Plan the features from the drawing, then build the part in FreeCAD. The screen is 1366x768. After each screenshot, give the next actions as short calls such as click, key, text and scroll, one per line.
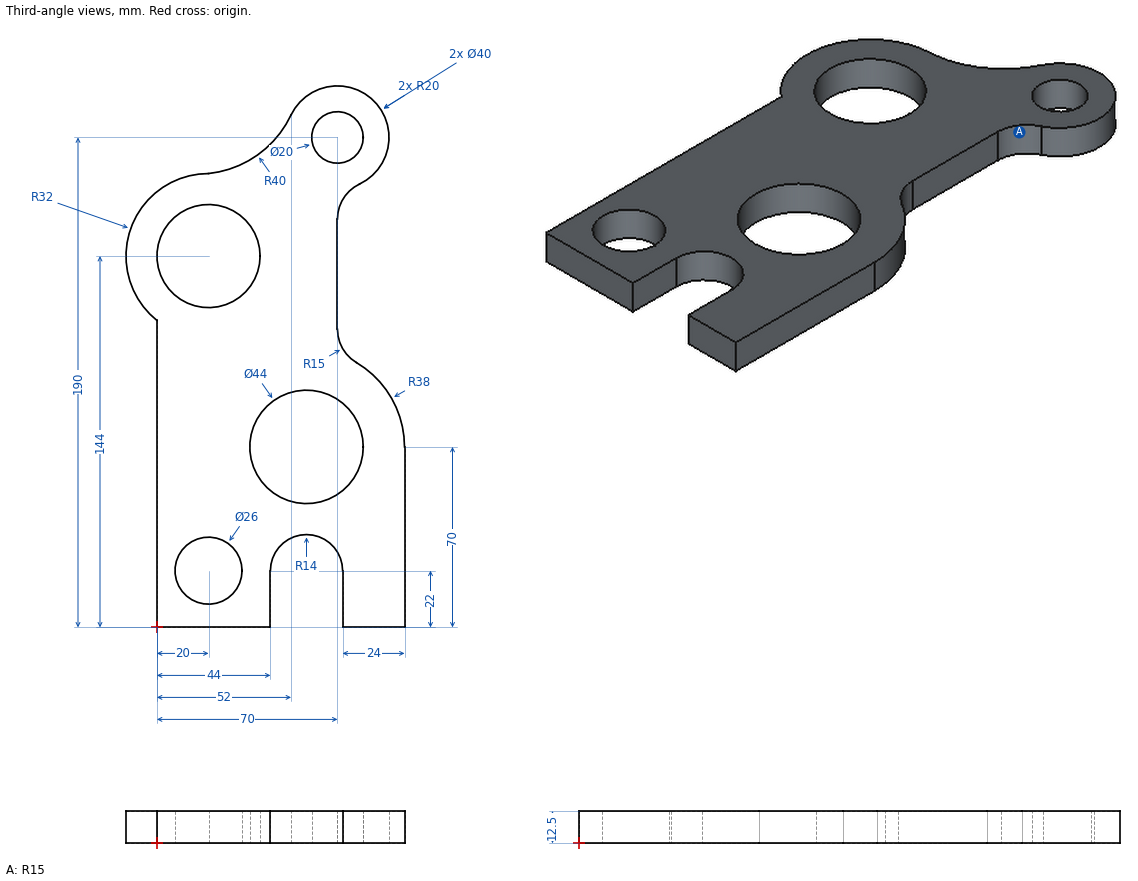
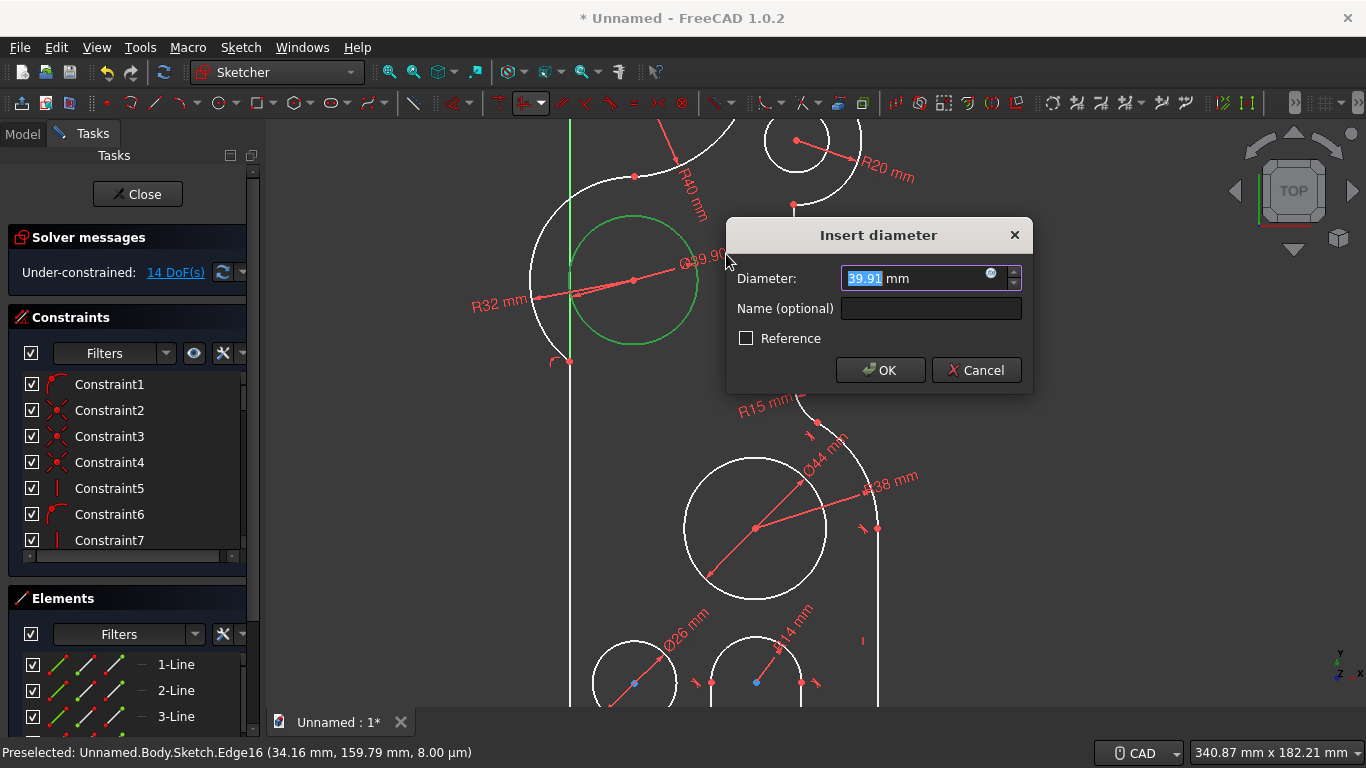
text(40)
key(Return)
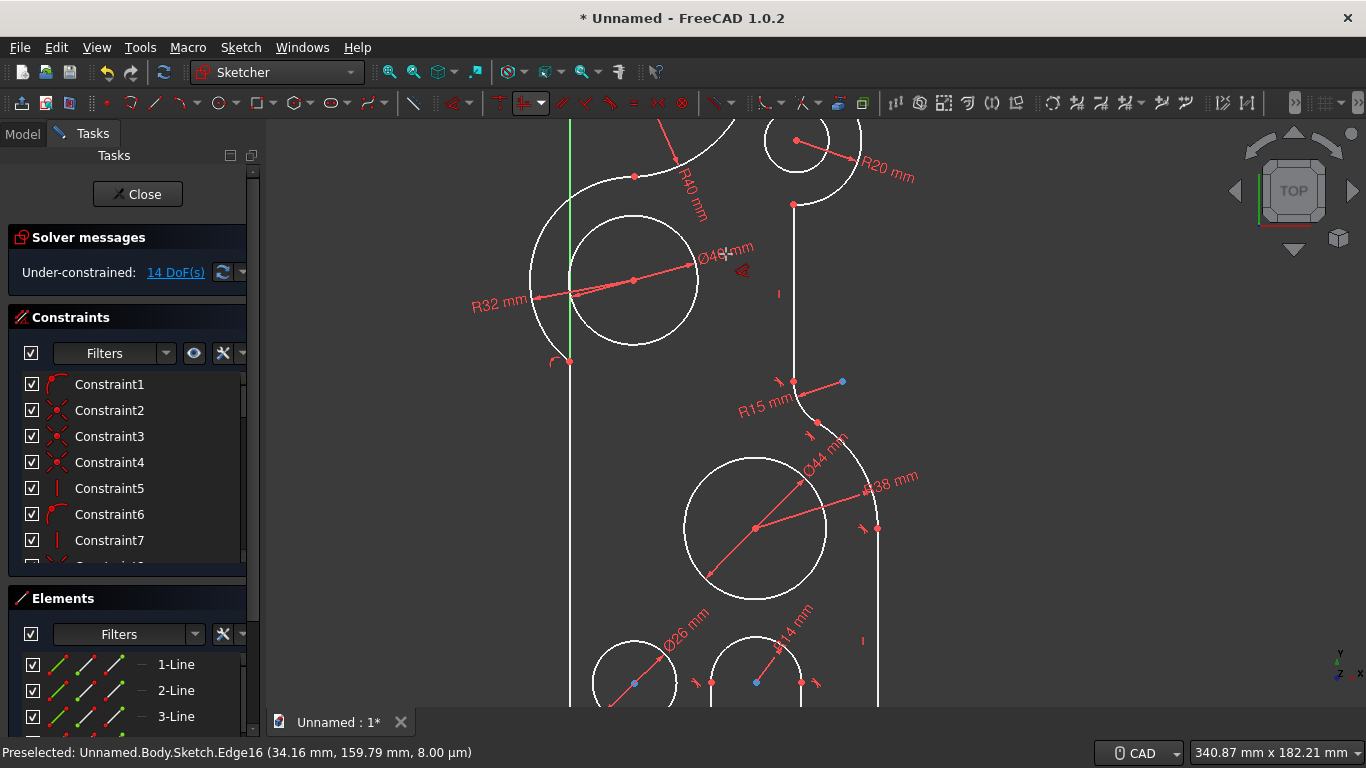
click(774, 163)
click(735, 158)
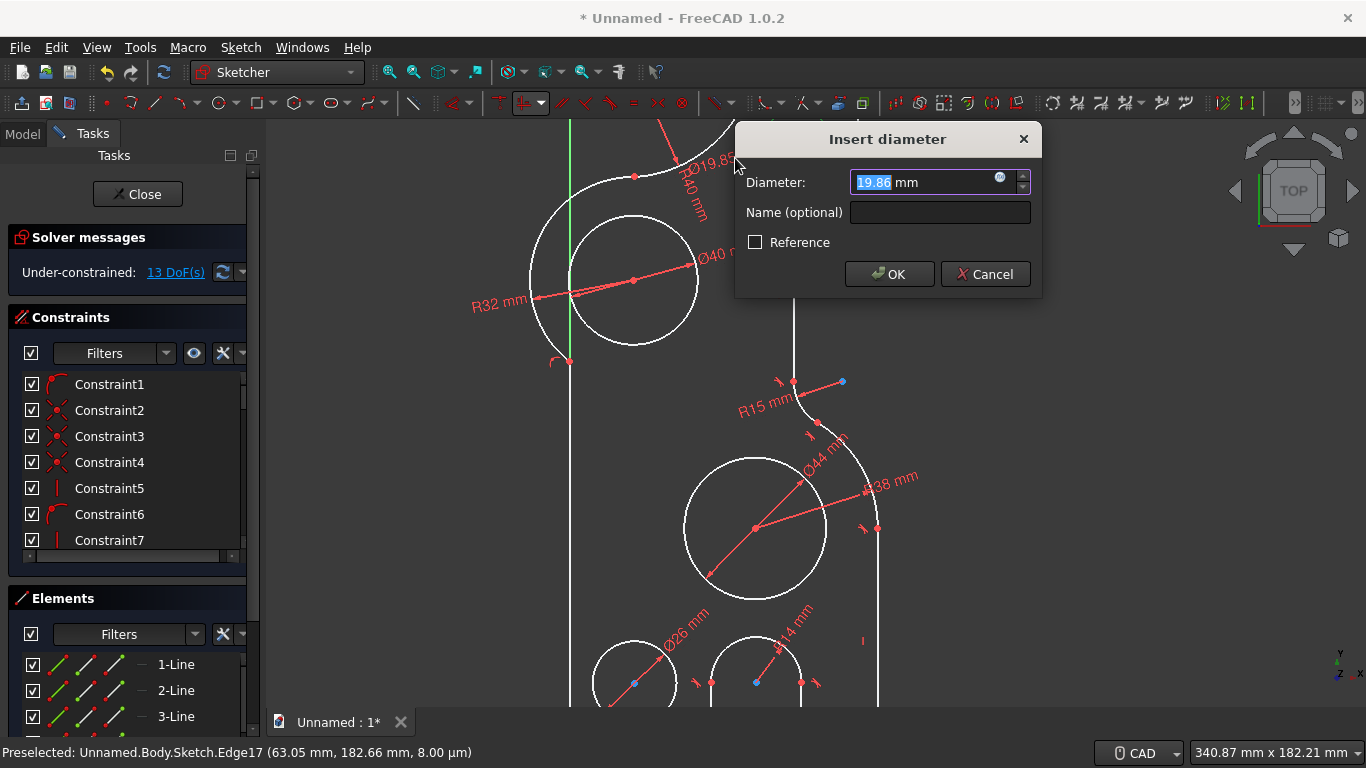
text(20)
key(Return)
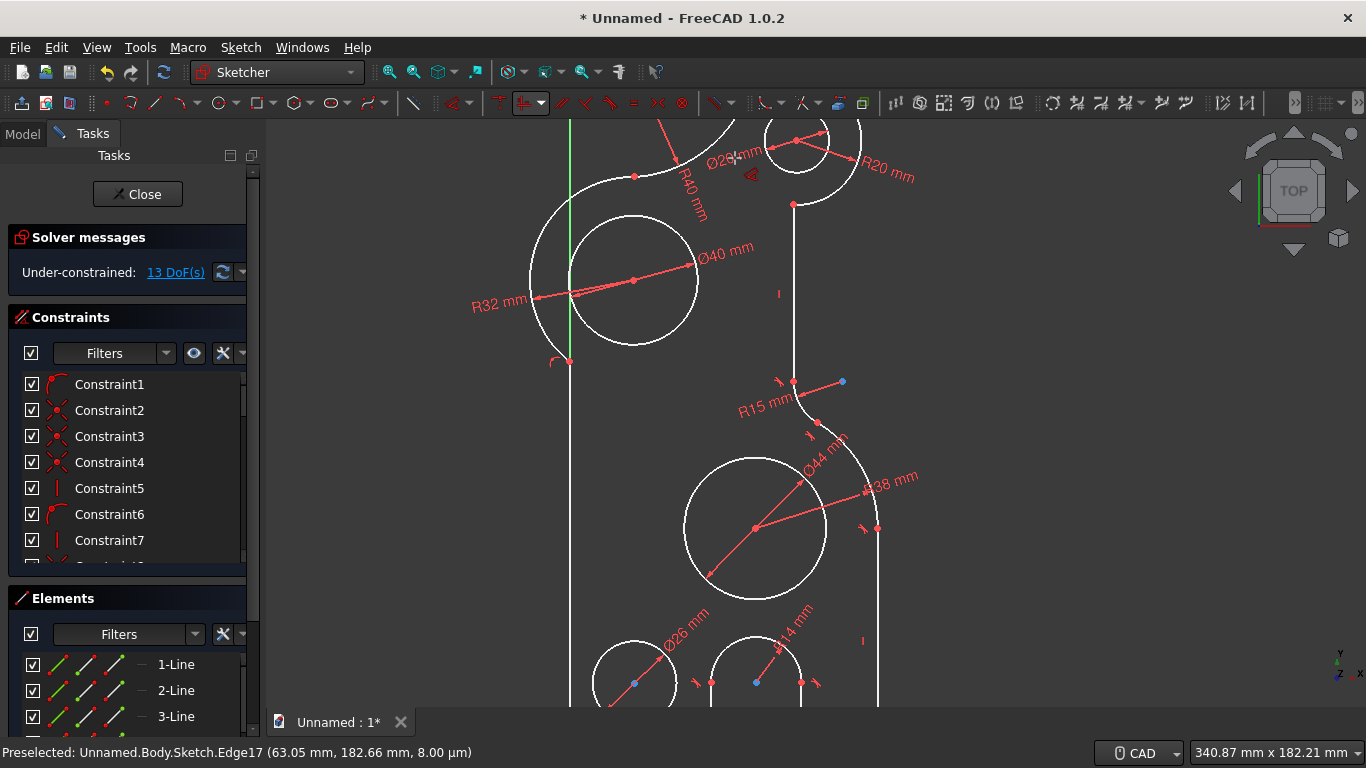
scroll(795, 395, down, 3)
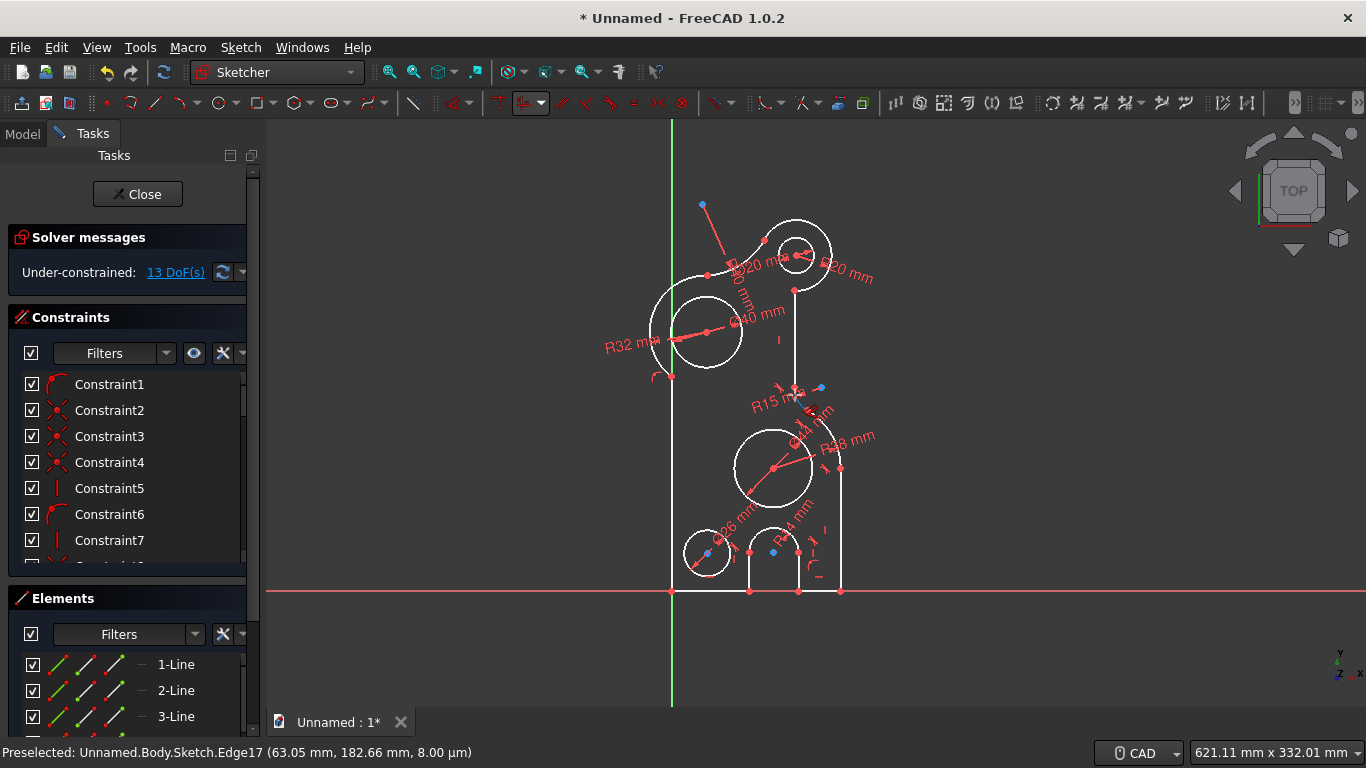
click(695, 591)
click(710, 625)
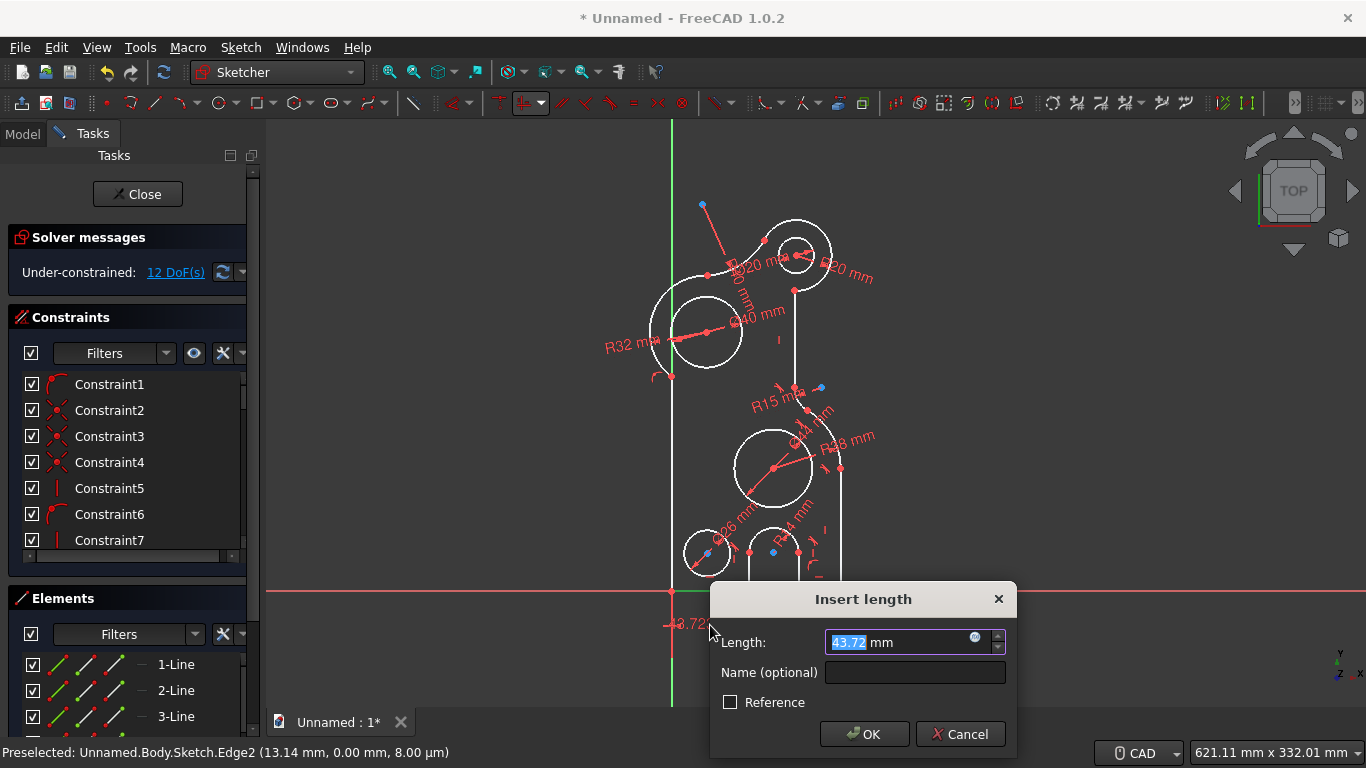
text(44)
key(Return)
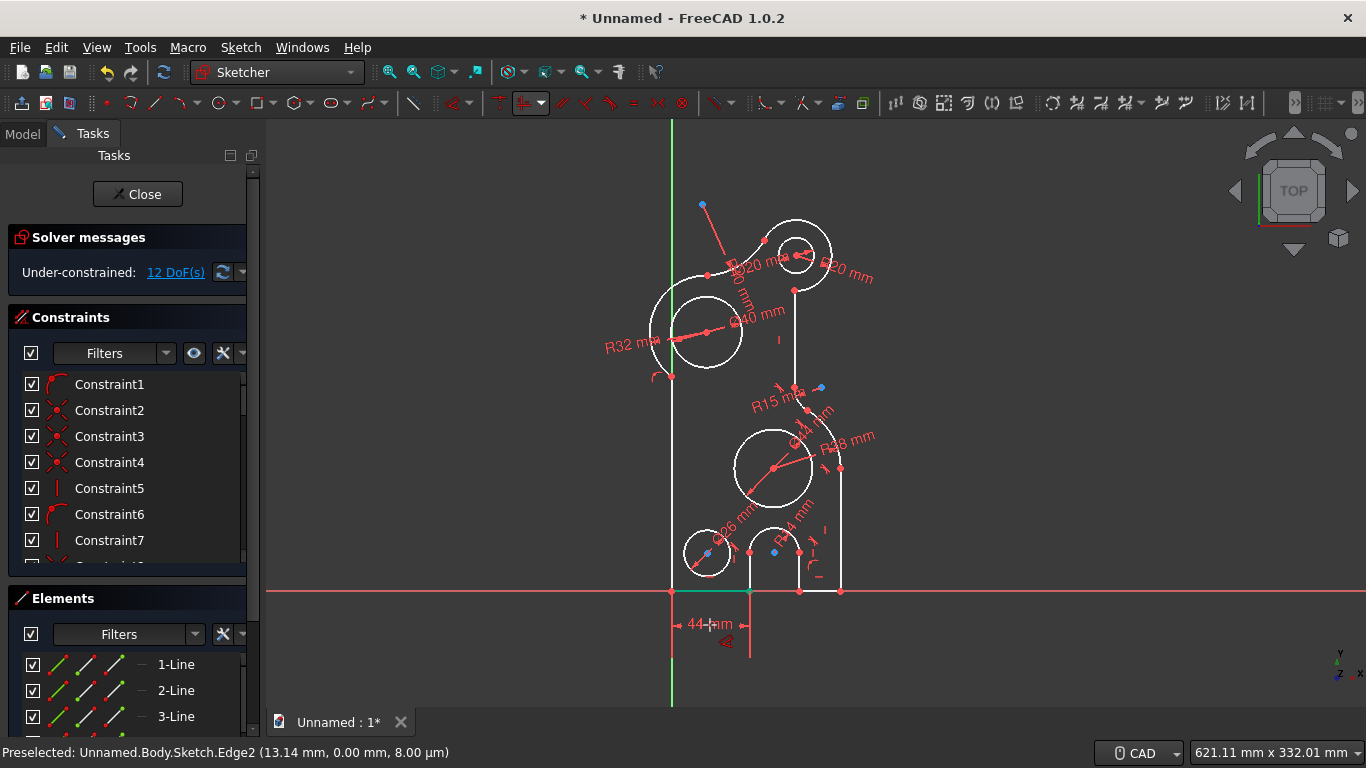
click(750, 580)
click(784, 572)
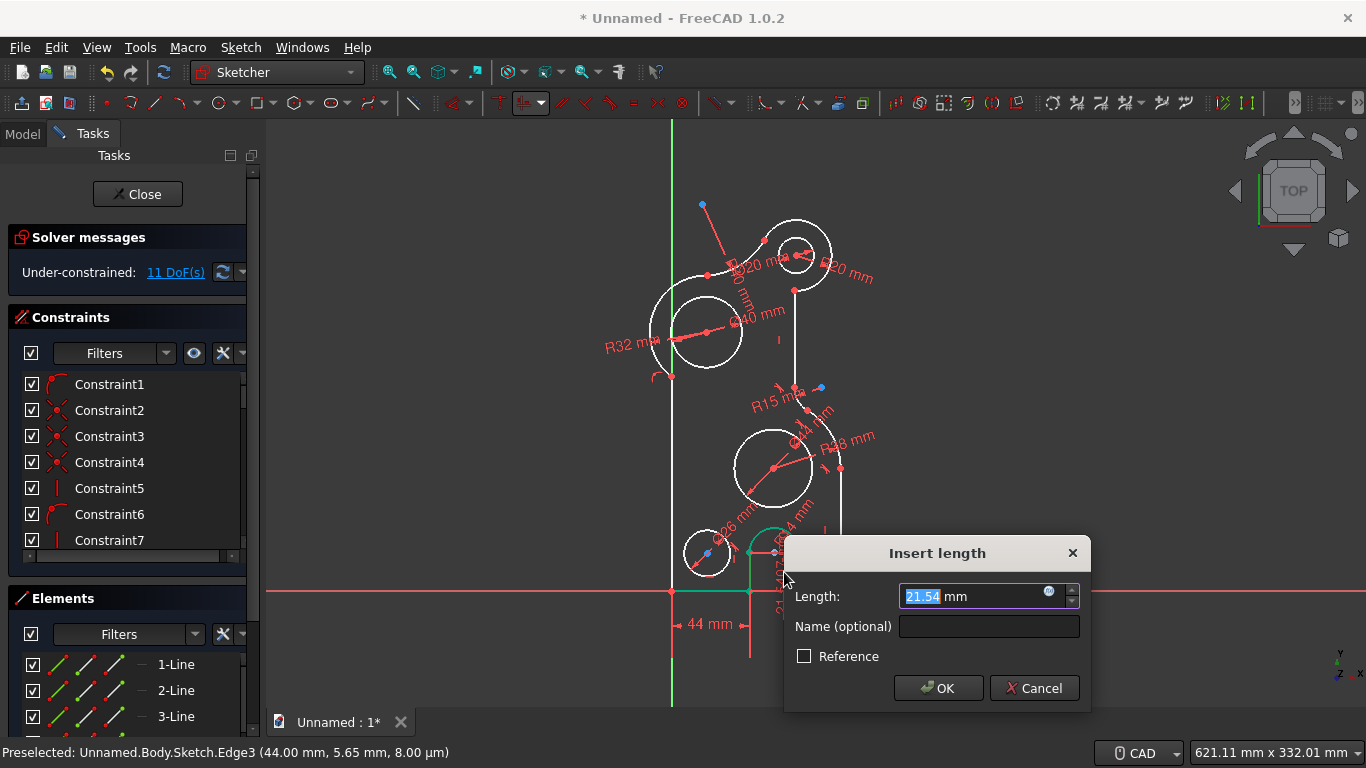
text(22)
key(Return)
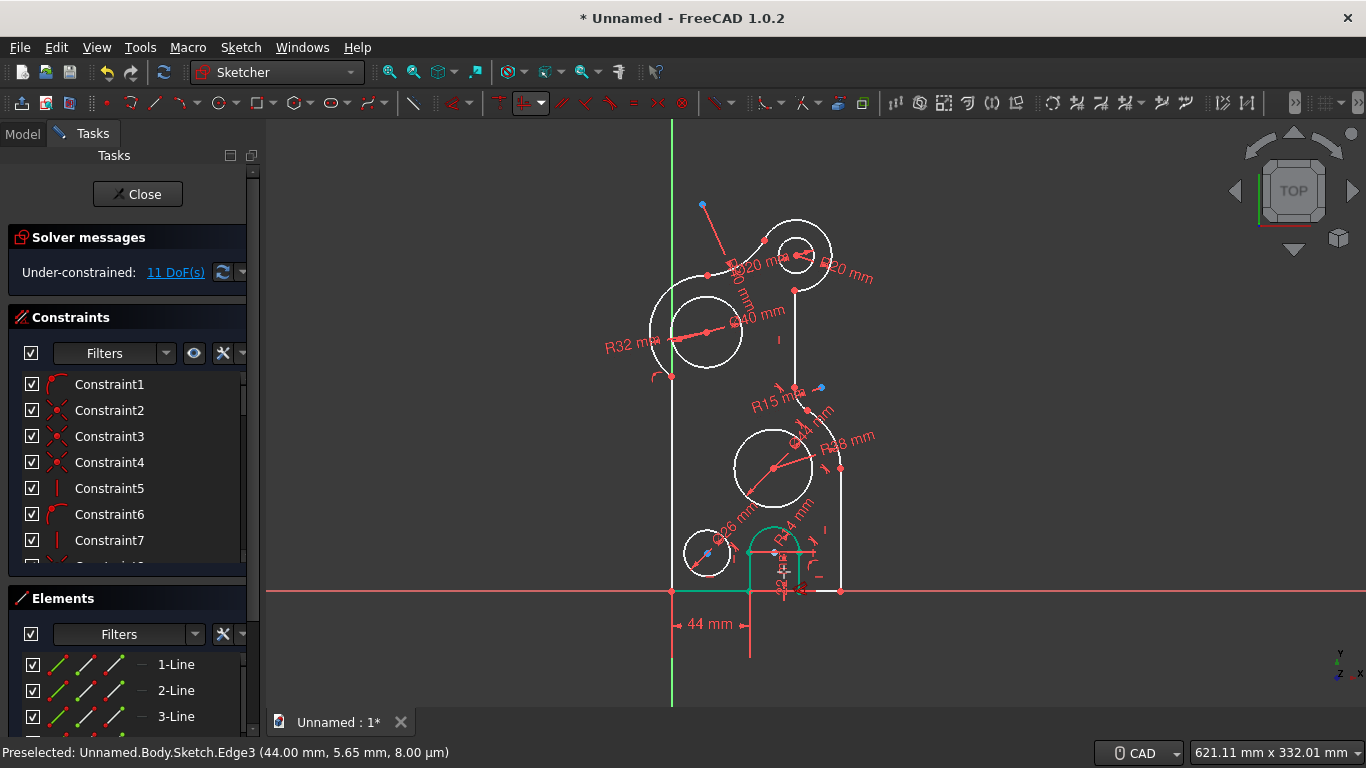
click(812, 591)
click(820, 625)